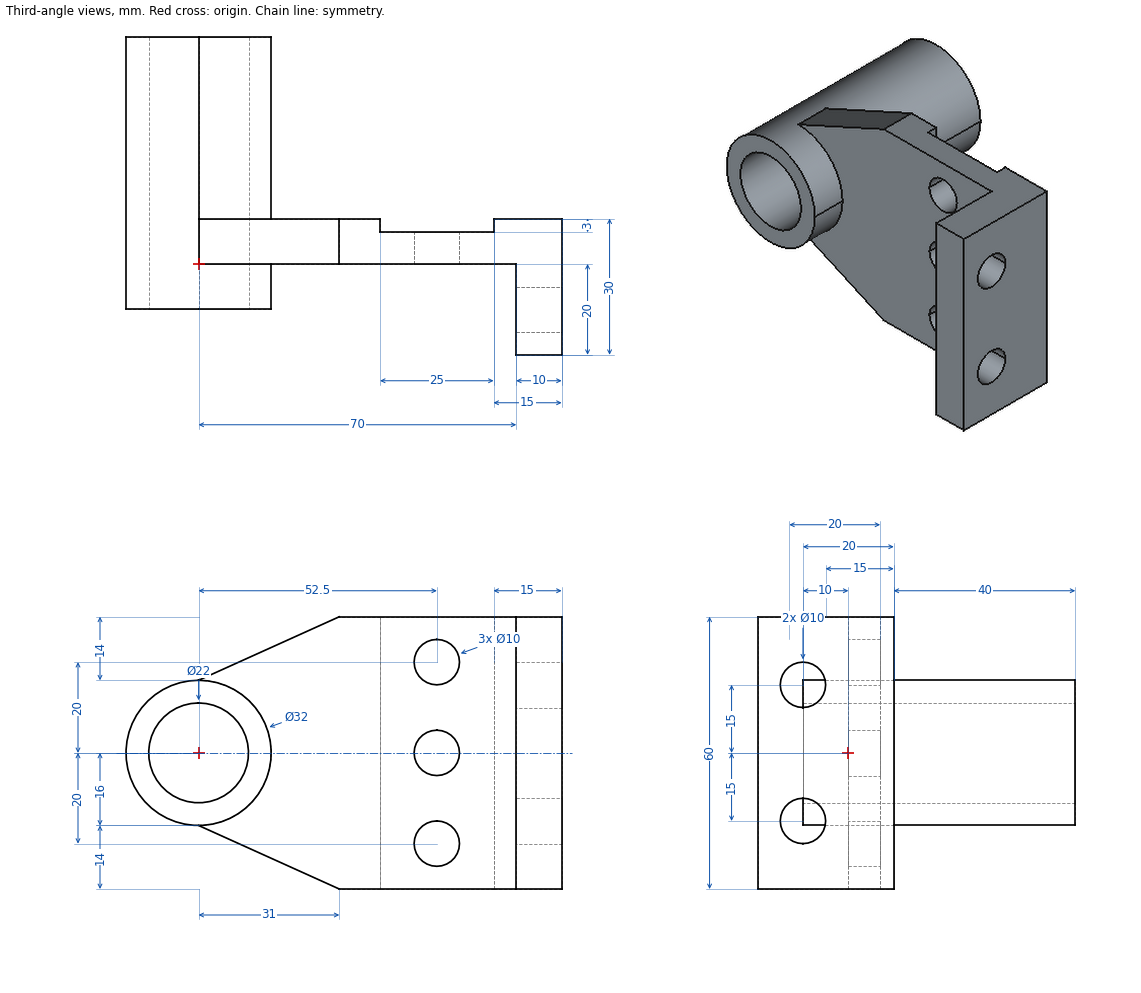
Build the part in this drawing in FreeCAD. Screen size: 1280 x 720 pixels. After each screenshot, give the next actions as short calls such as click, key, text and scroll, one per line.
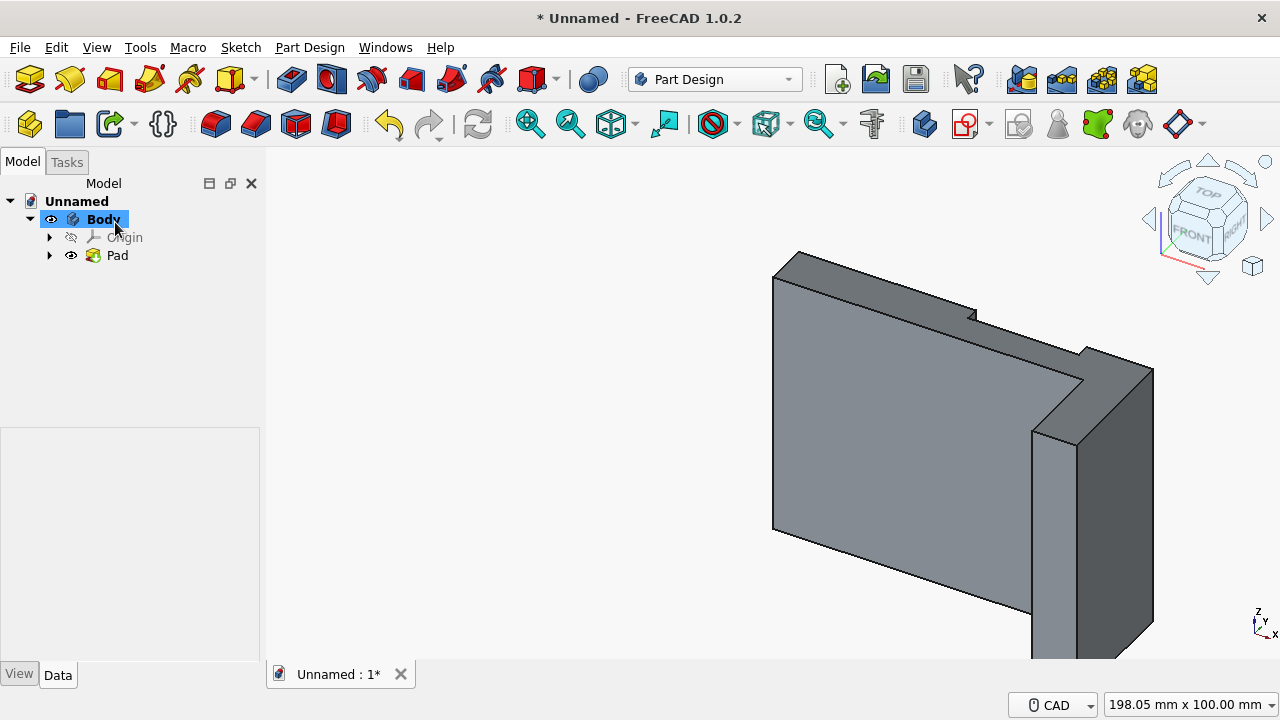
click(532, 124)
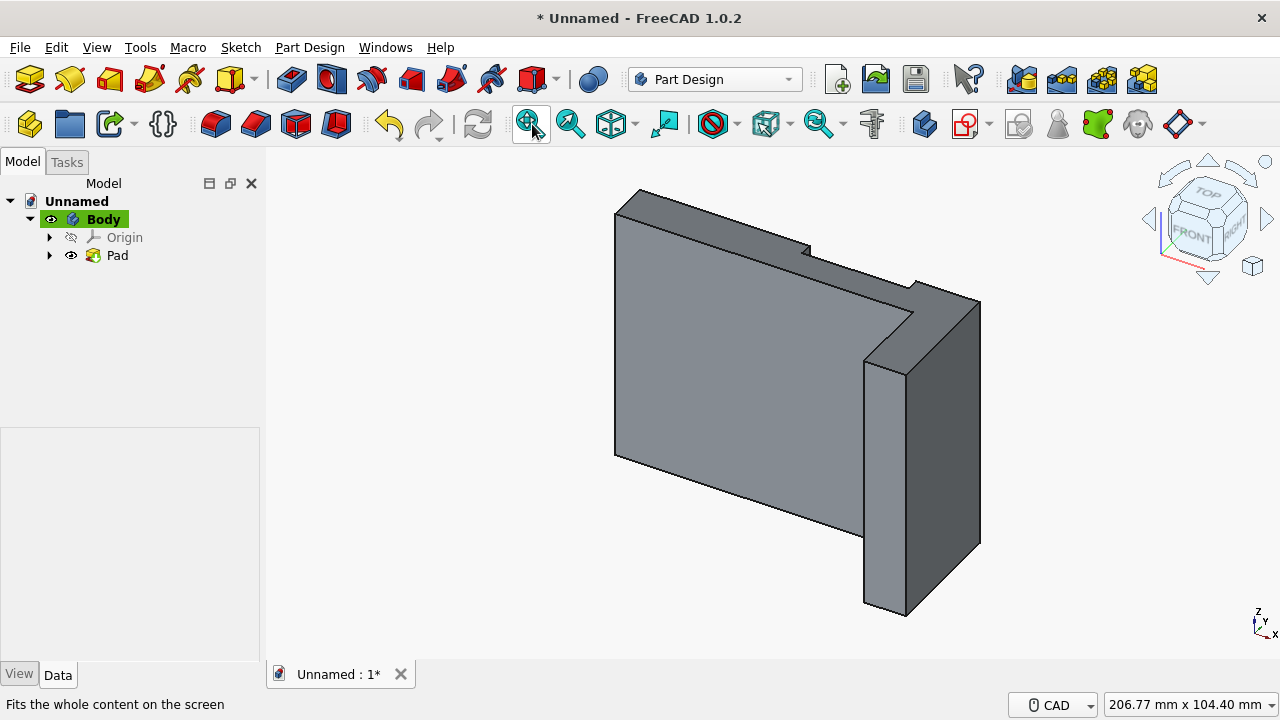
click(943, 424)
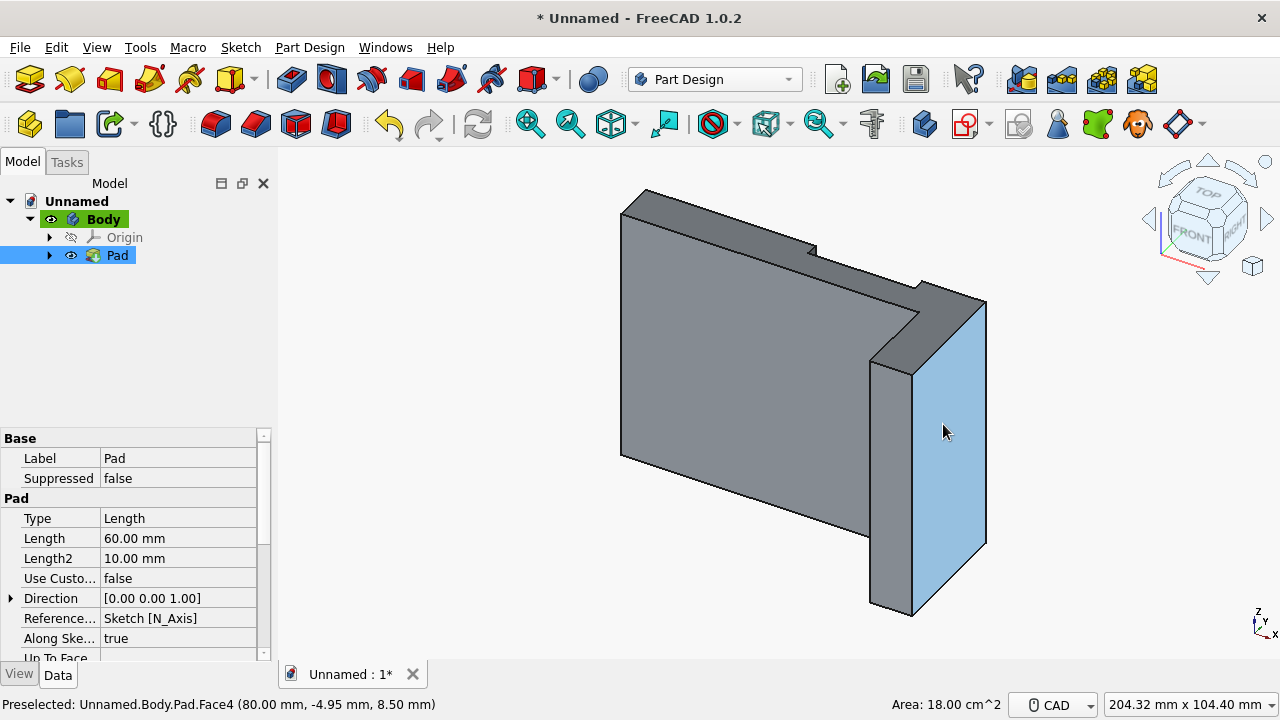
click(966, 124)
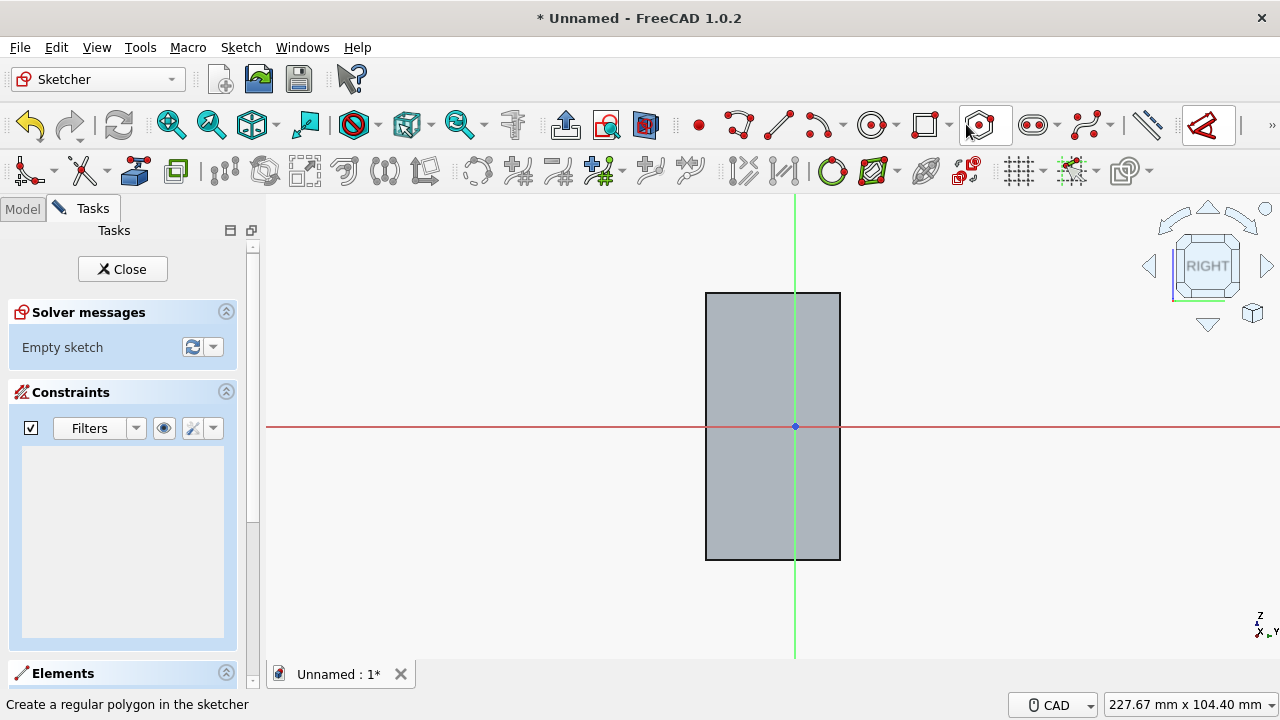
scroll(879, 426, up, 2)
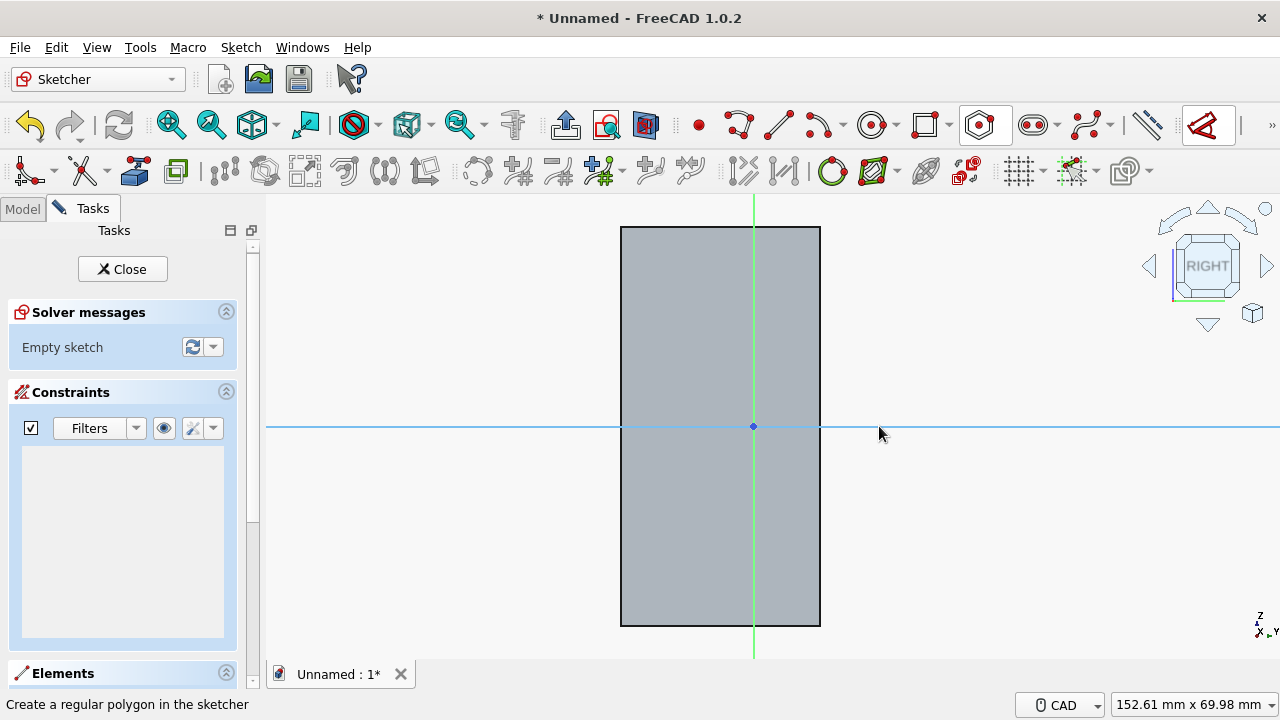
click(872, 126)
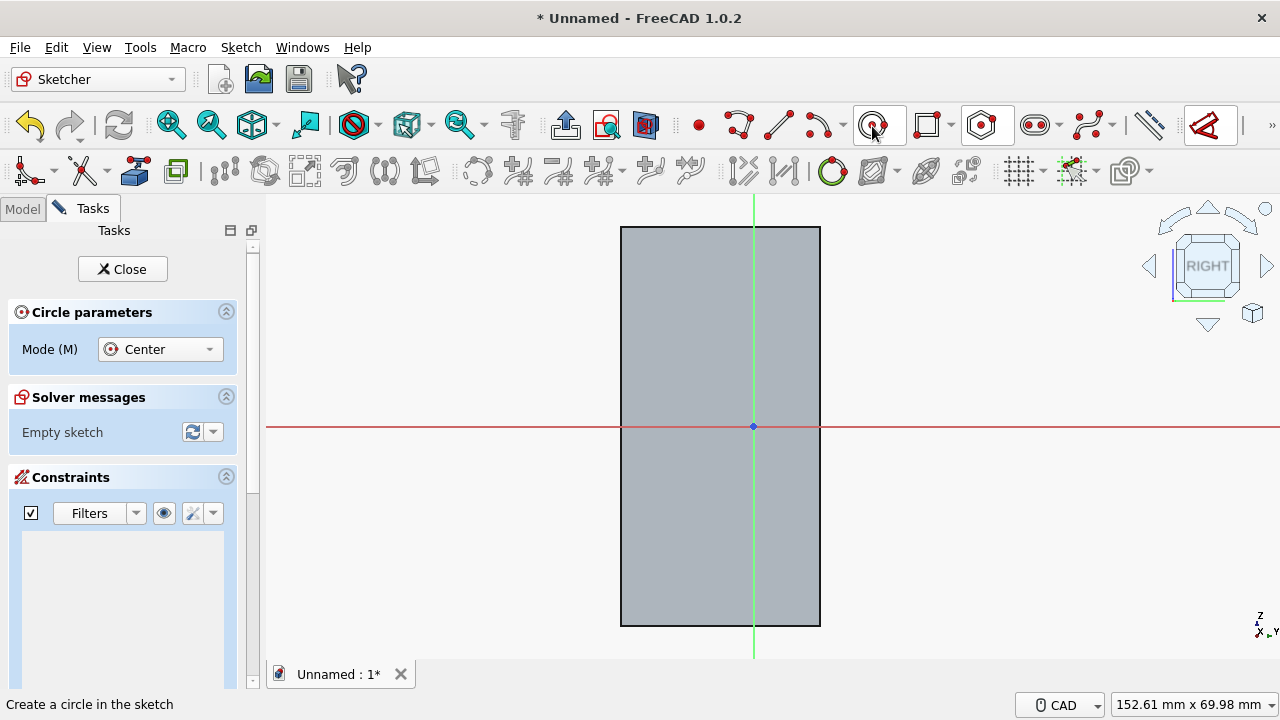
click(687, 327)
move(711, 303)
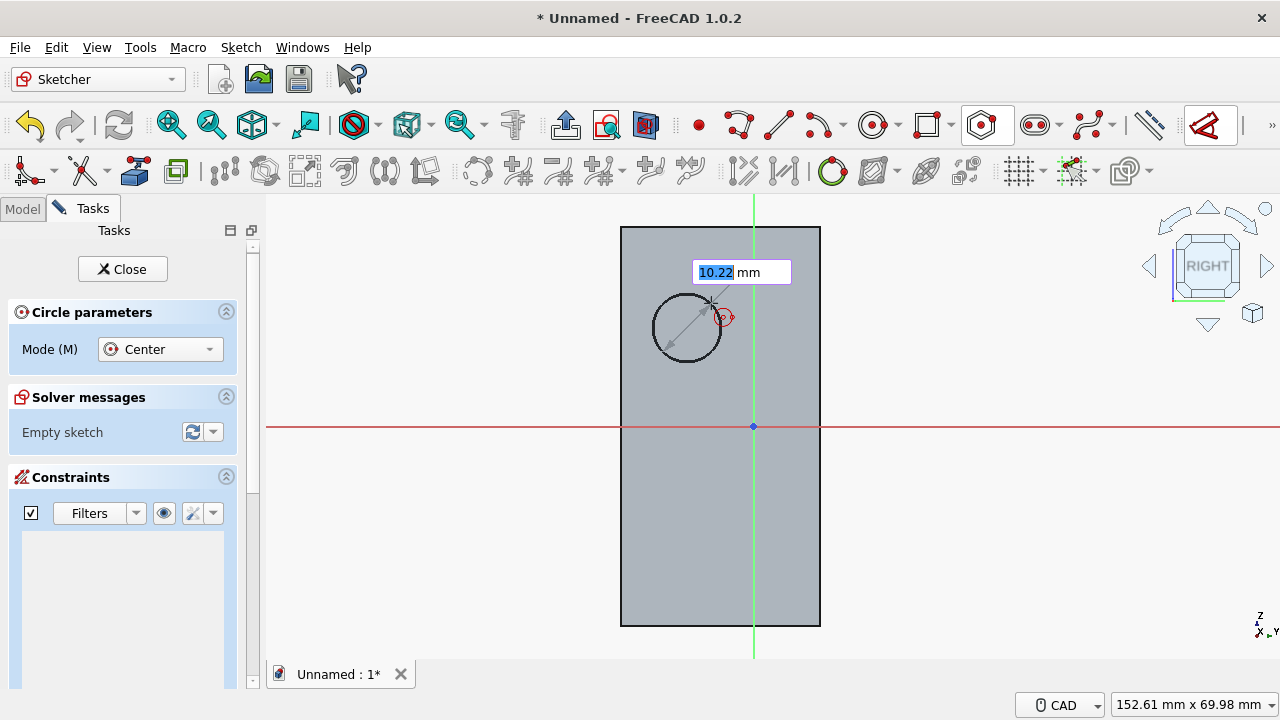
text(10)
key(Return)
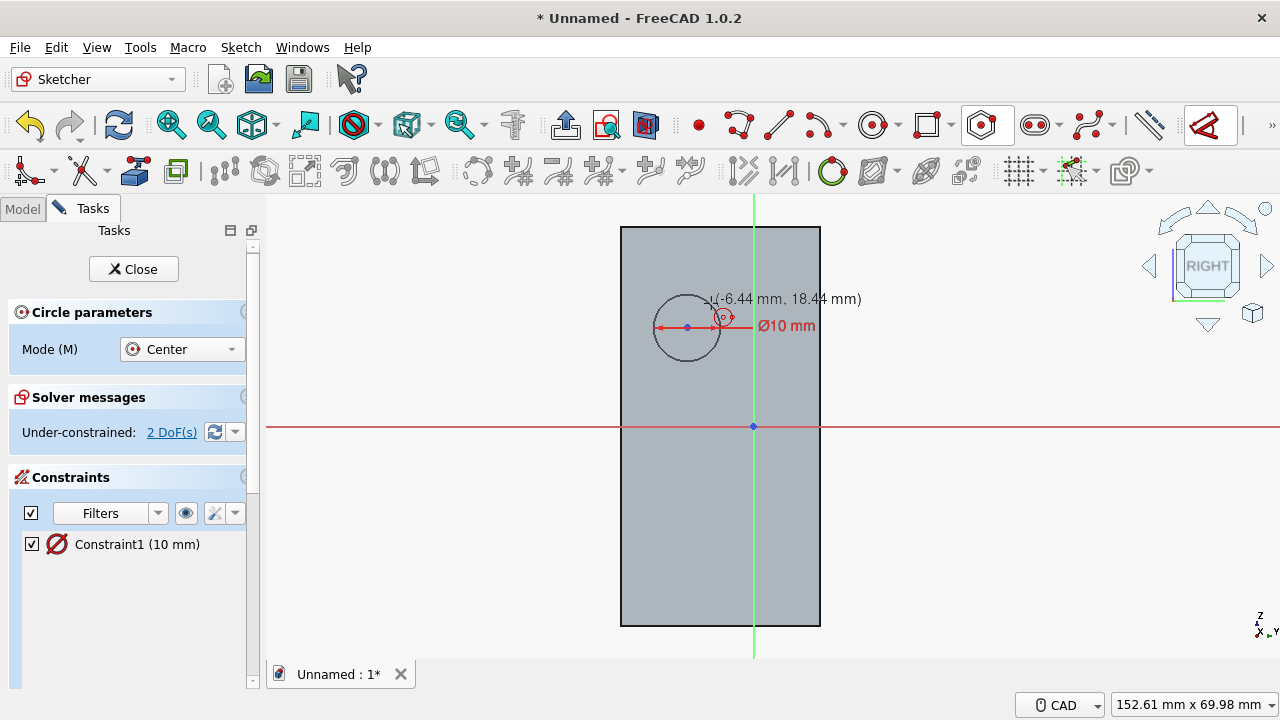
click(687, 526)
move(711, 503)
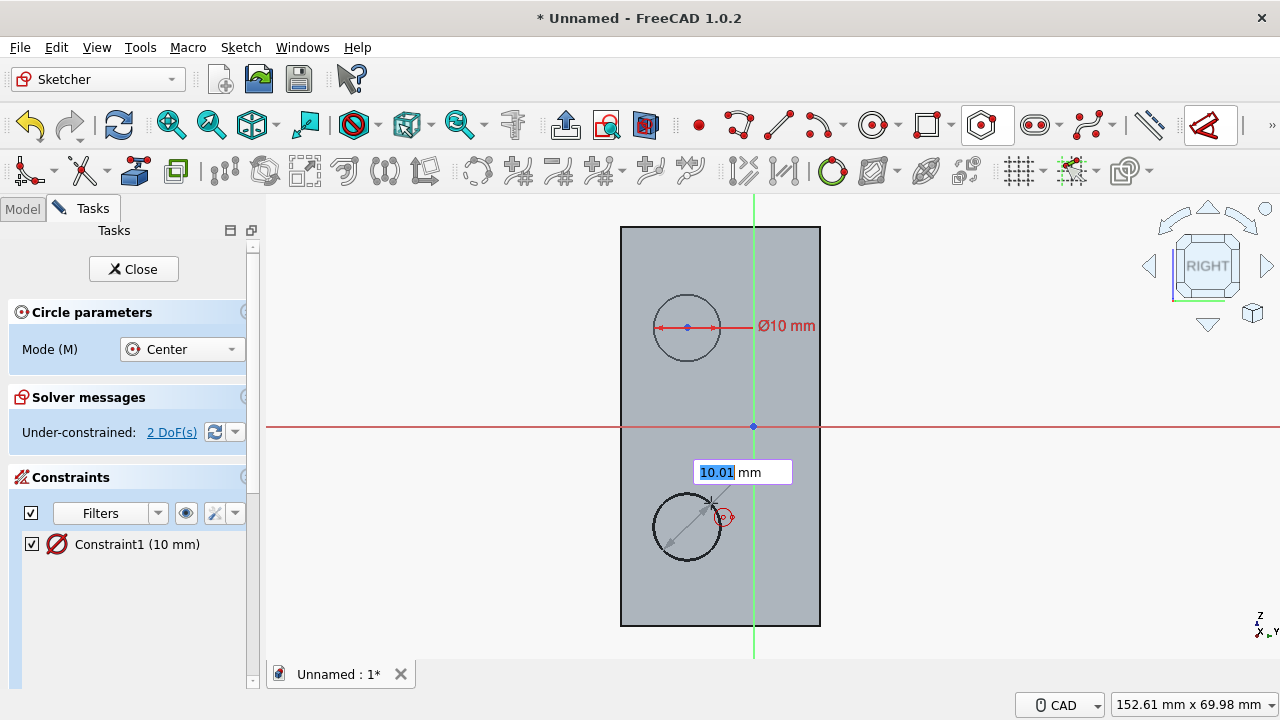
text(10)
key(Return)
key(Escape)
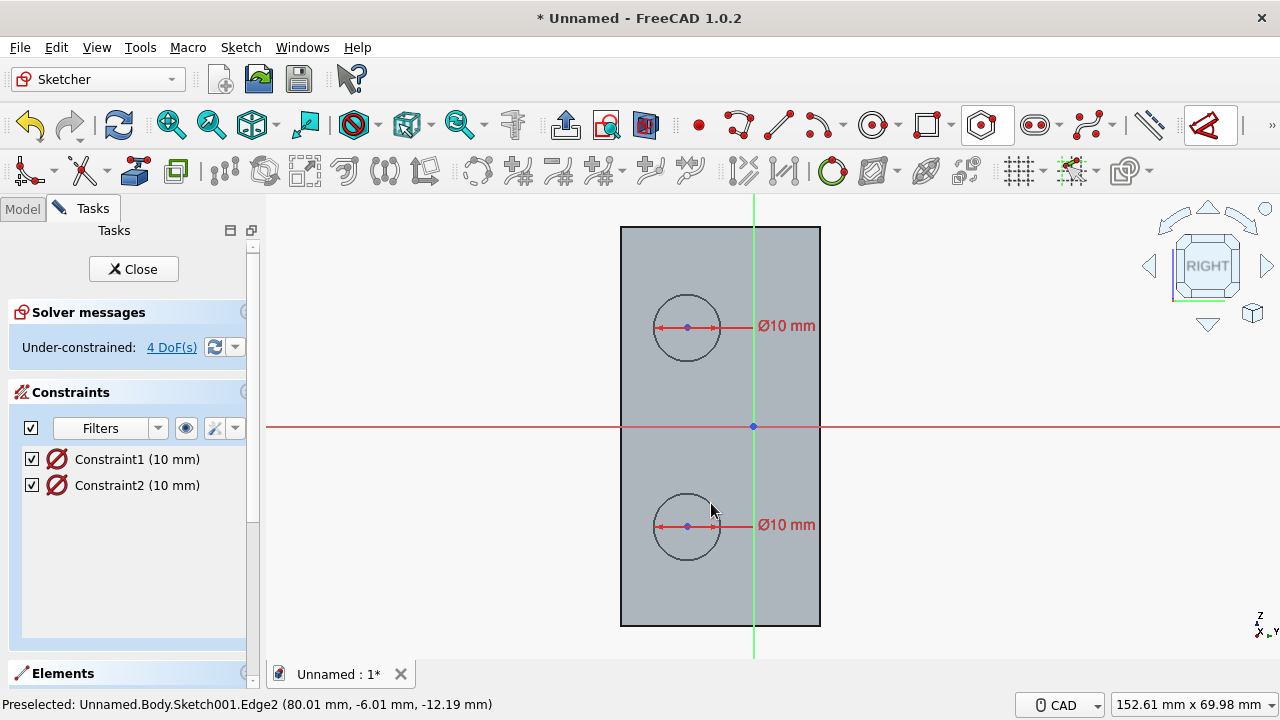
click(687, 328)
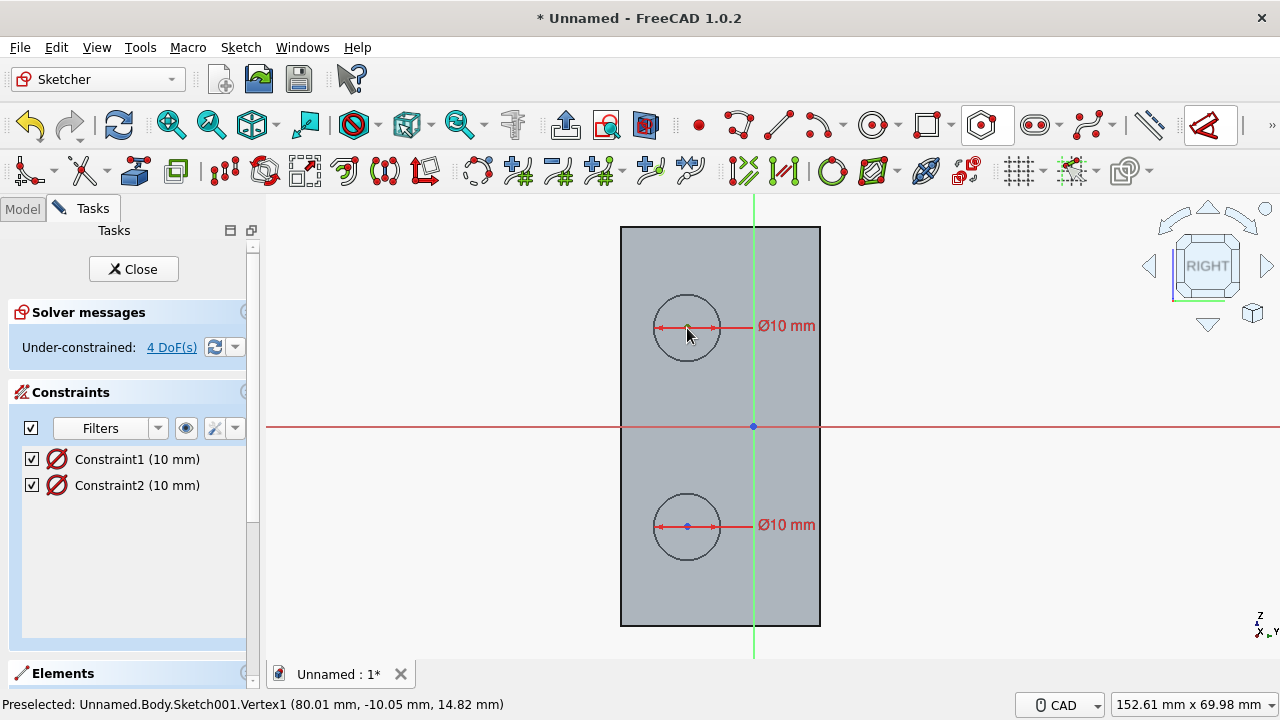
click(687, 527)